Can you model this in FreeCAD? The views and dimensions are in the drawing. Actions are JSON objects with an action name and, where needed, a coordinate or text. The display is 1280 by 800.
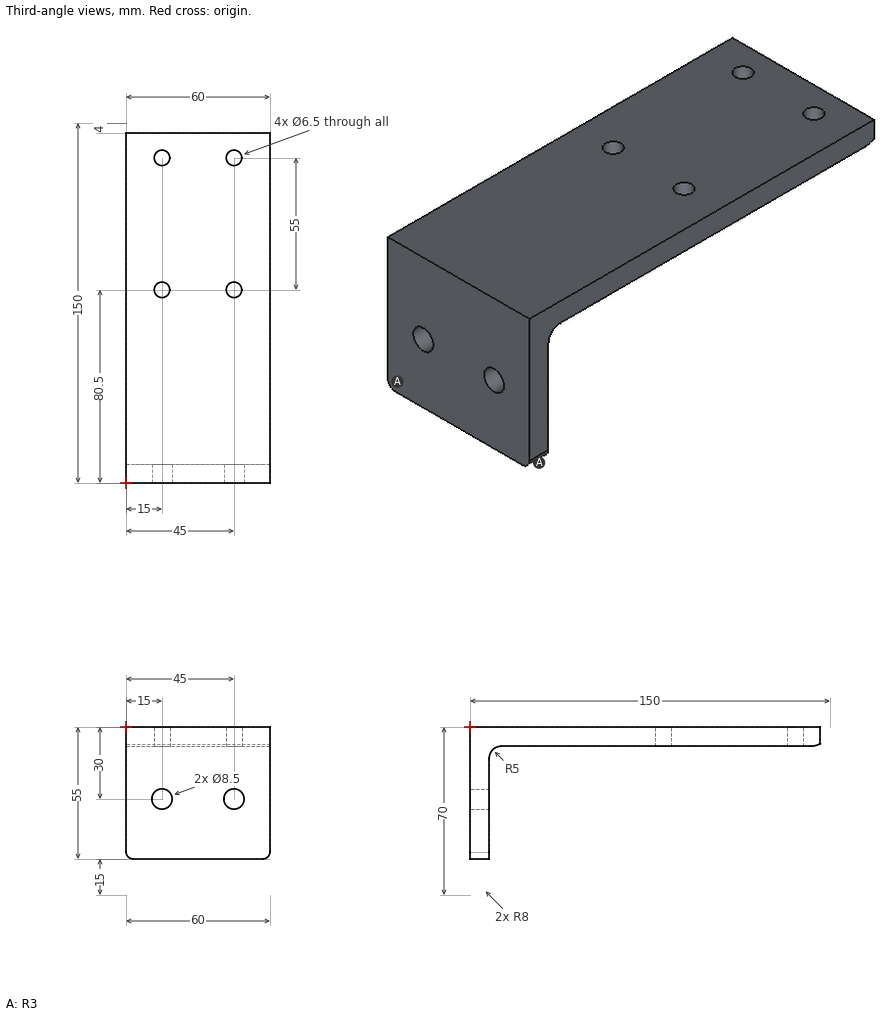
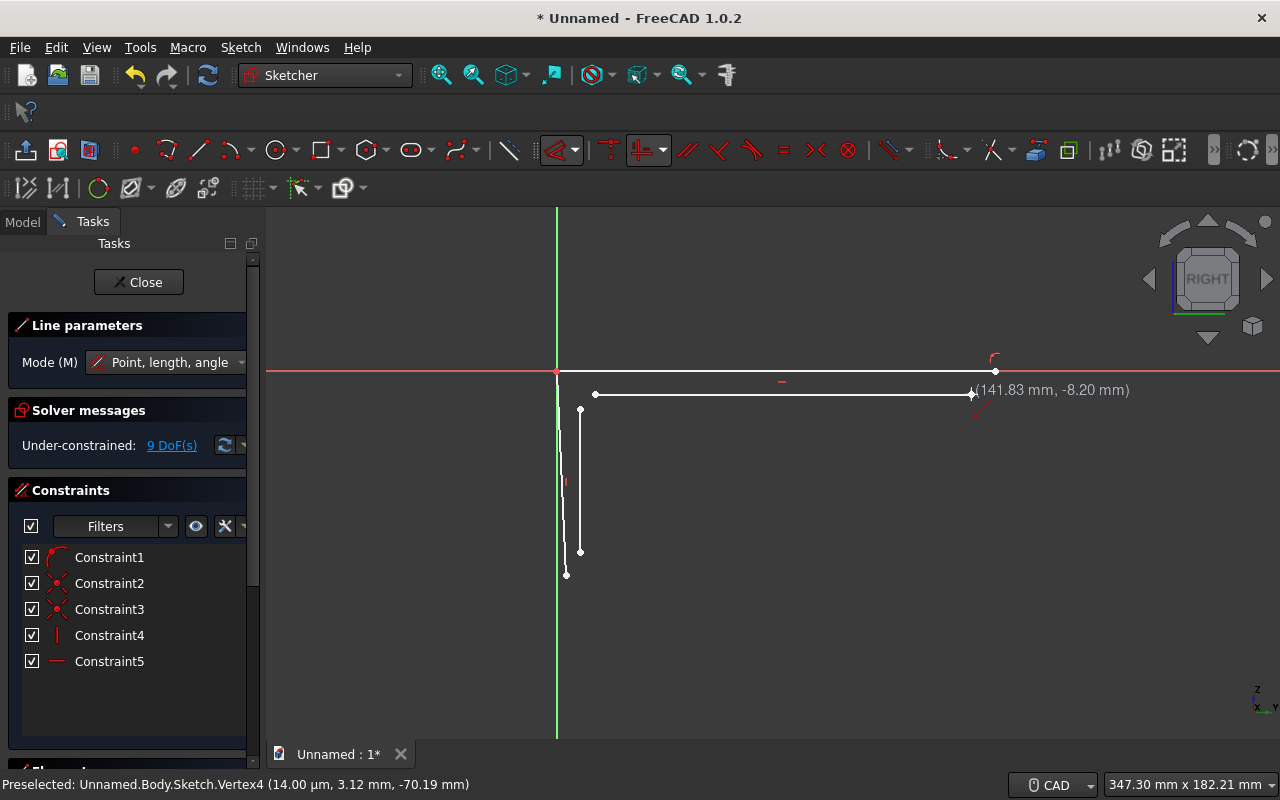
{"action": "key", "text": "g 3 a"}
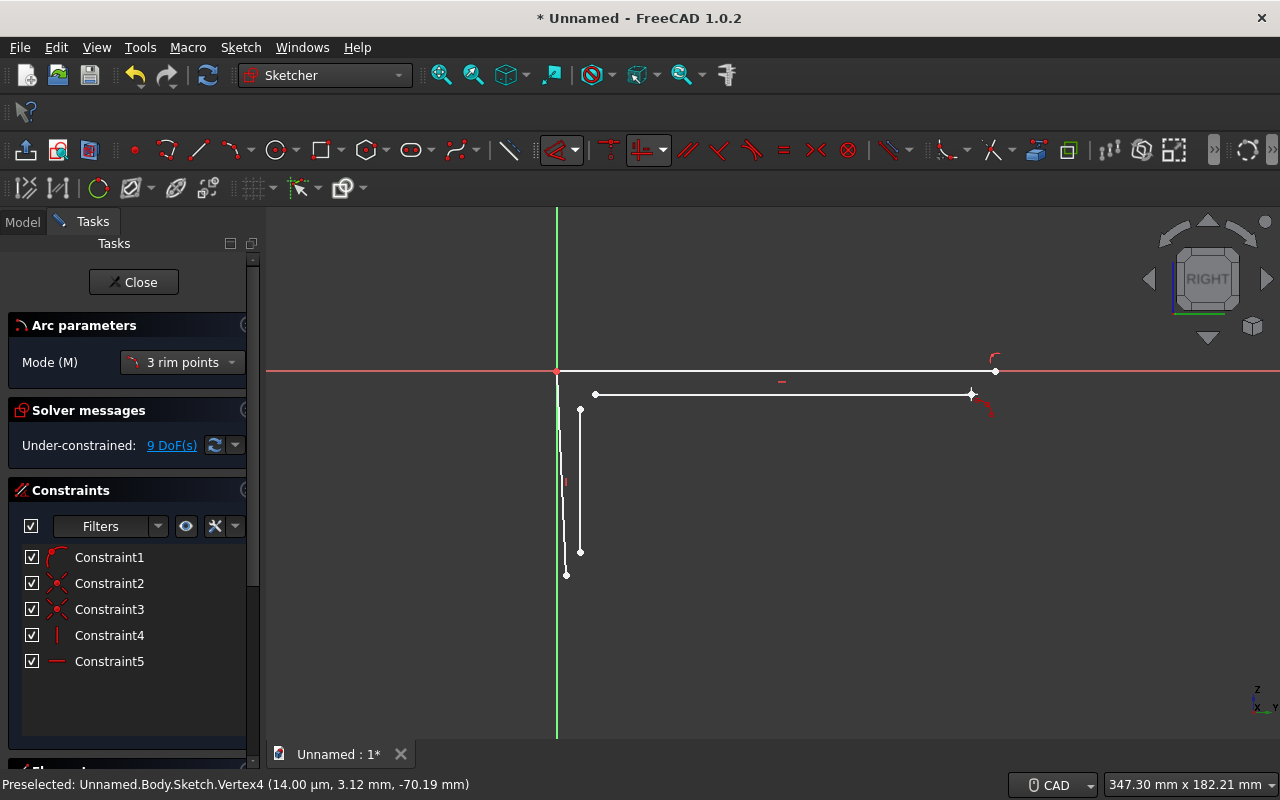
{"action": "left_click", "coordinate": [566, 576]}
{"action": "left_click", "coordinate": [580, 553]}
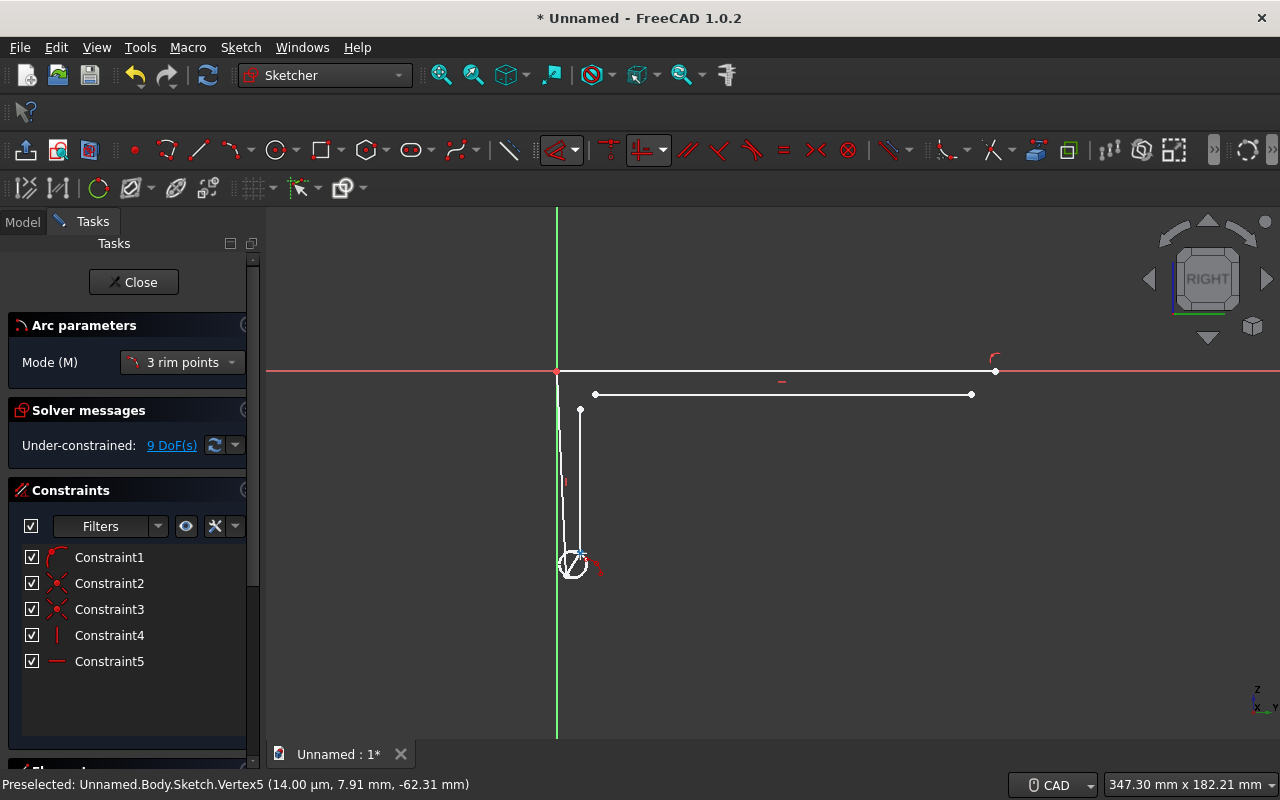
{"action": "scroll", "coordinate": [573, 569], "scroll_direction": "up", "scroll_amount": 5}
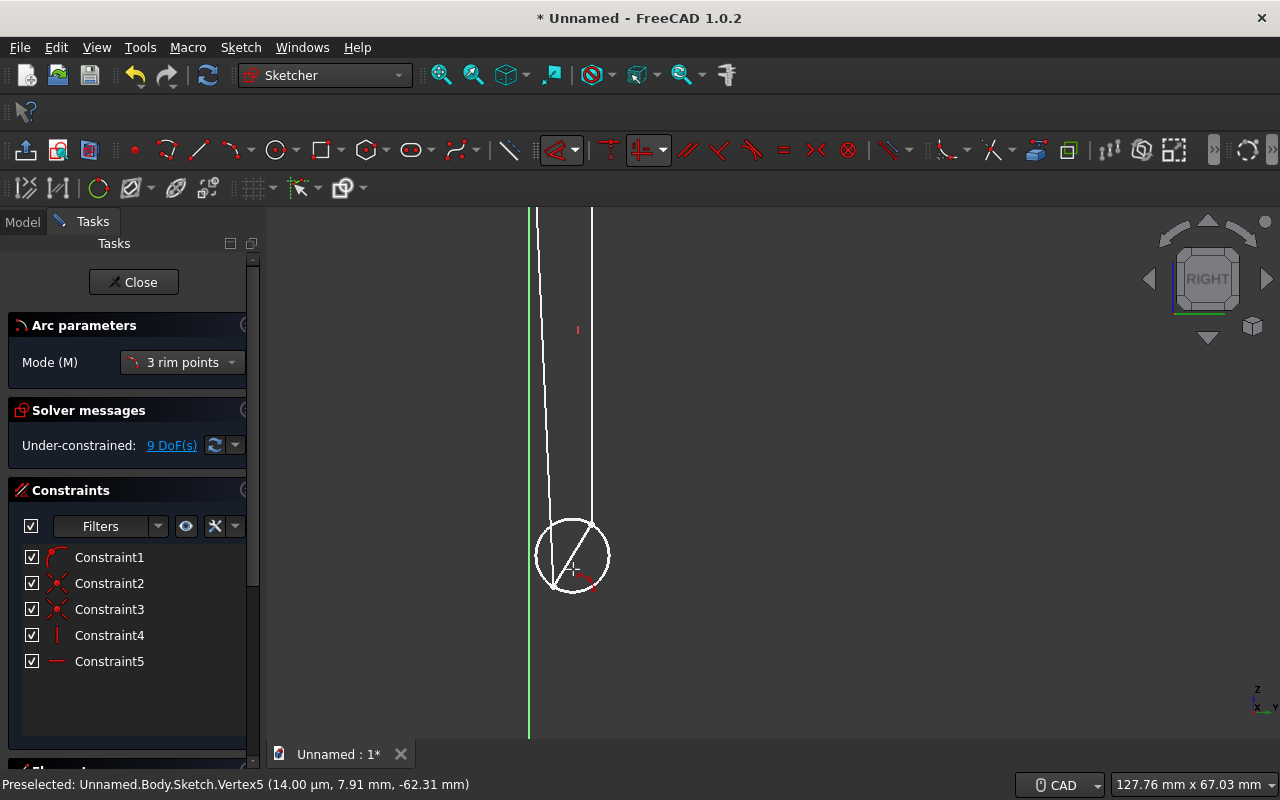
{"action": "left_click", "coordinate": [574, 567]}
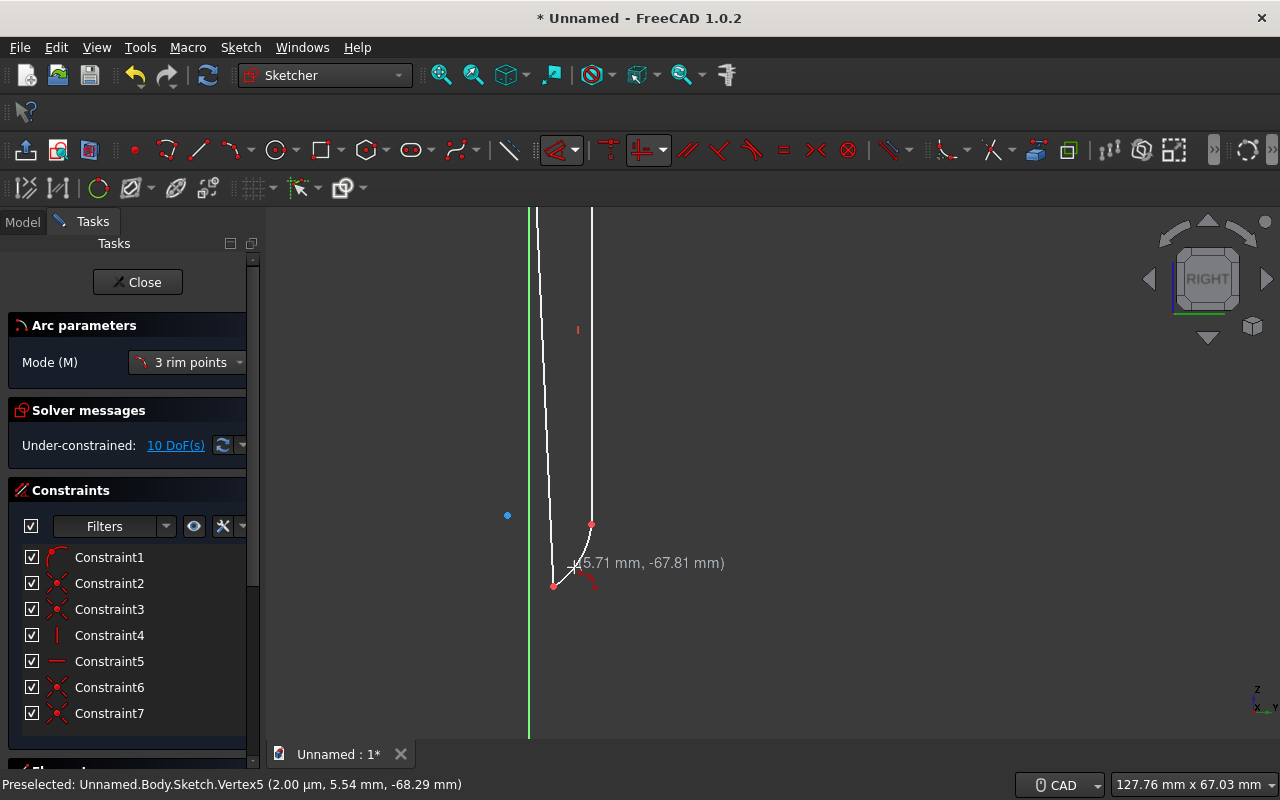
{"action": "scroll", "coordinate": [362, 608], "scroll_direction": "down", "scroll_amount": 4}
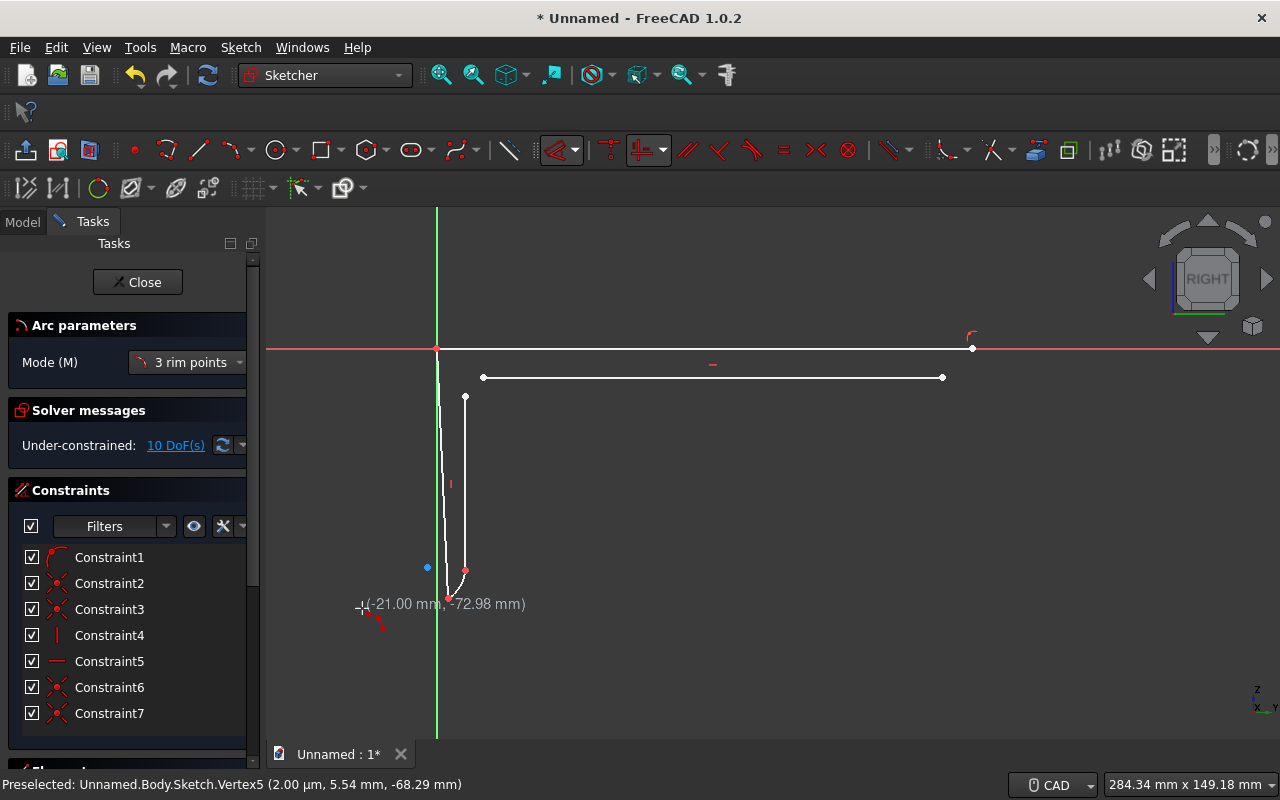
{"action": "left_click", "coordinate": [465, 396]}
{"action": "left_click", "coordinate": [483, 378]}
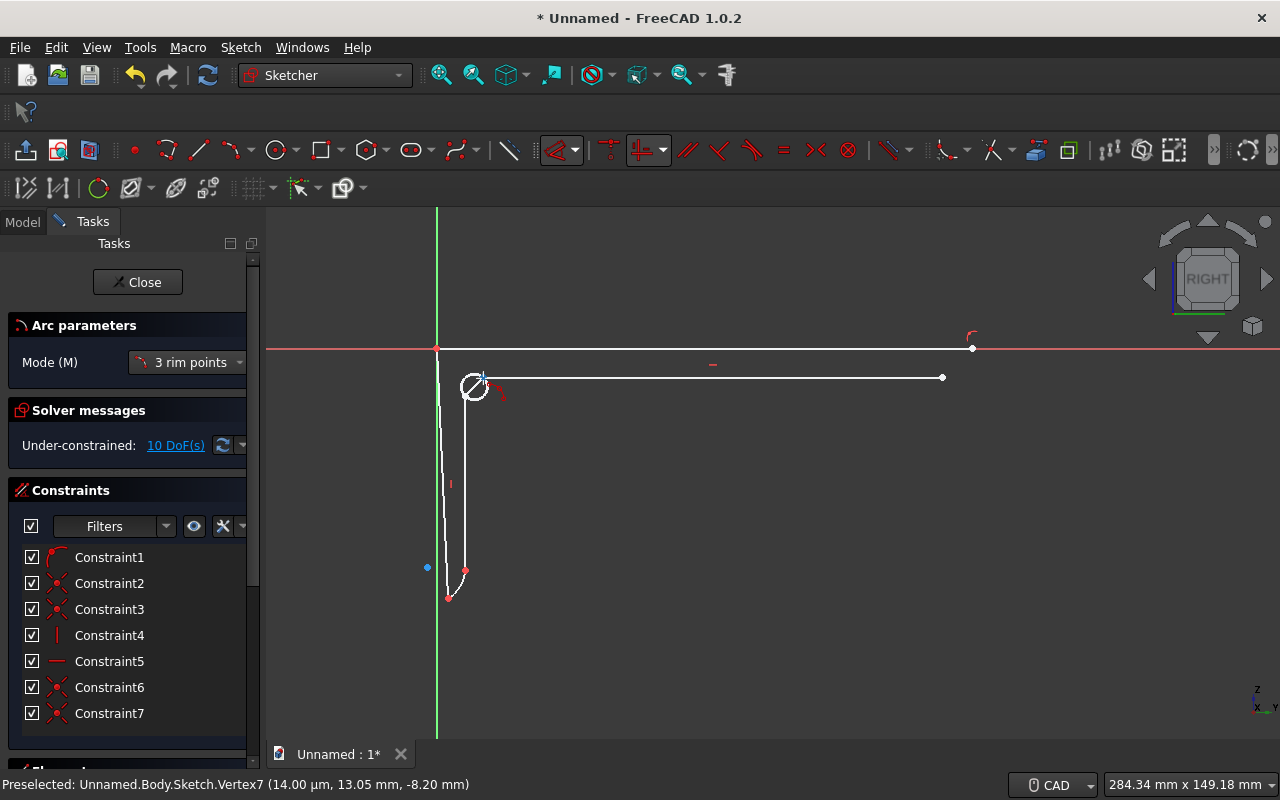
{"action": "scroll", "coordinate": [471, 382], "scroll_direction": "up", "scroll_amount": 6}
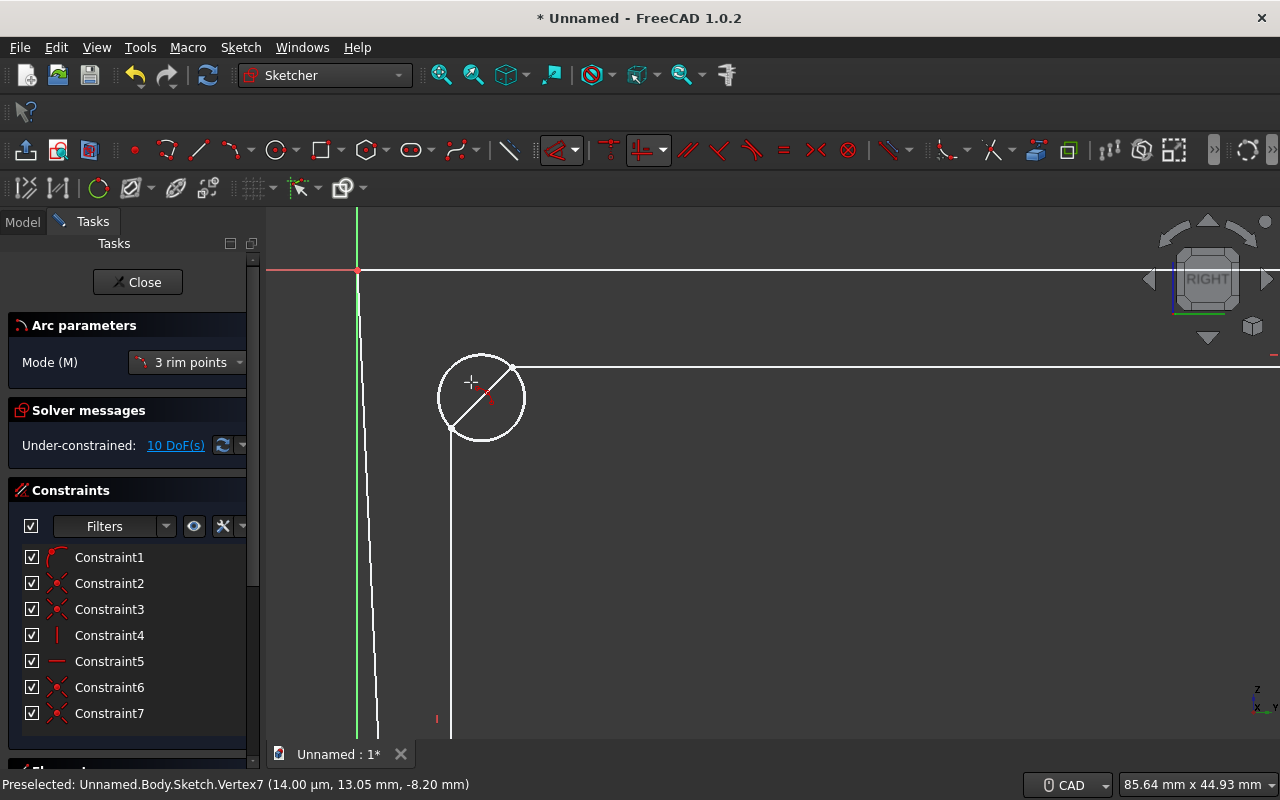
{"action": "left_click", "coordinate": [470, 382]}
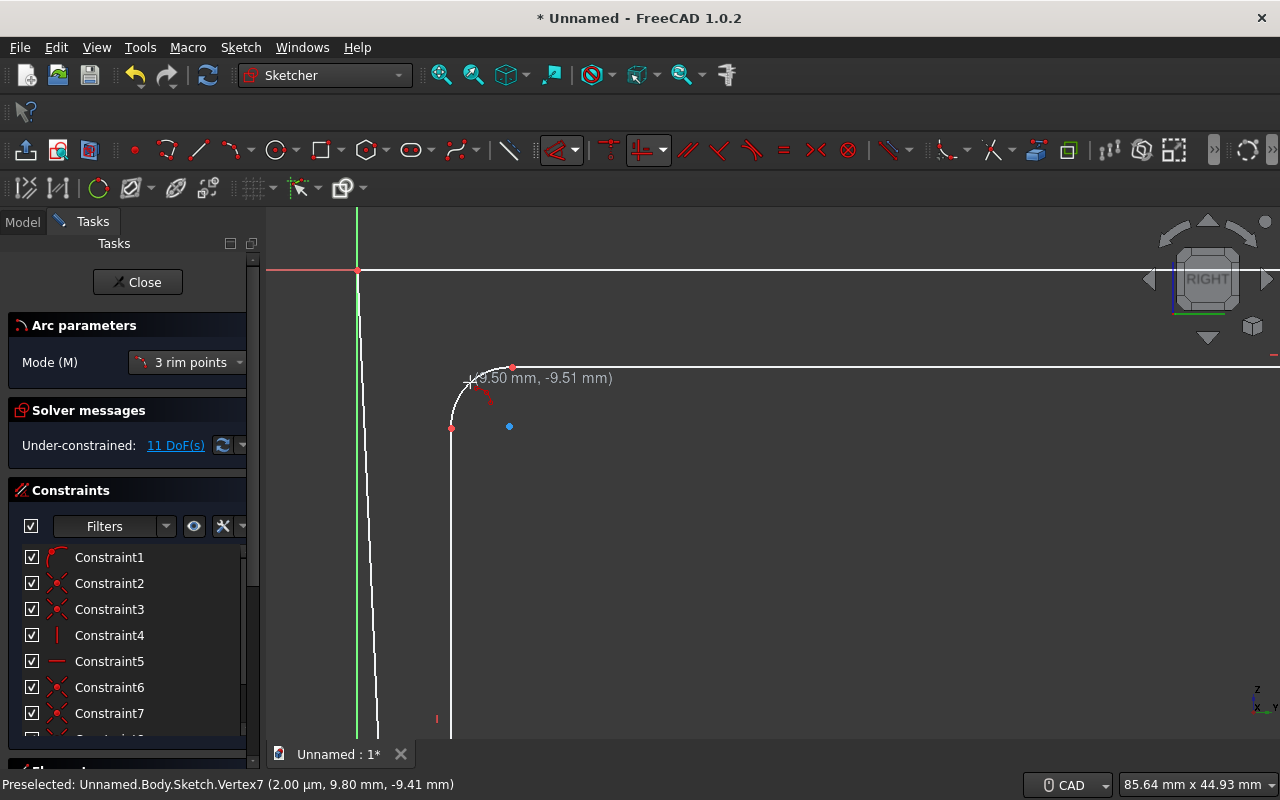
{"action": "scroll", "coordinate": [471, 382], "scroll_direction": "down", "scroll_amount": 6}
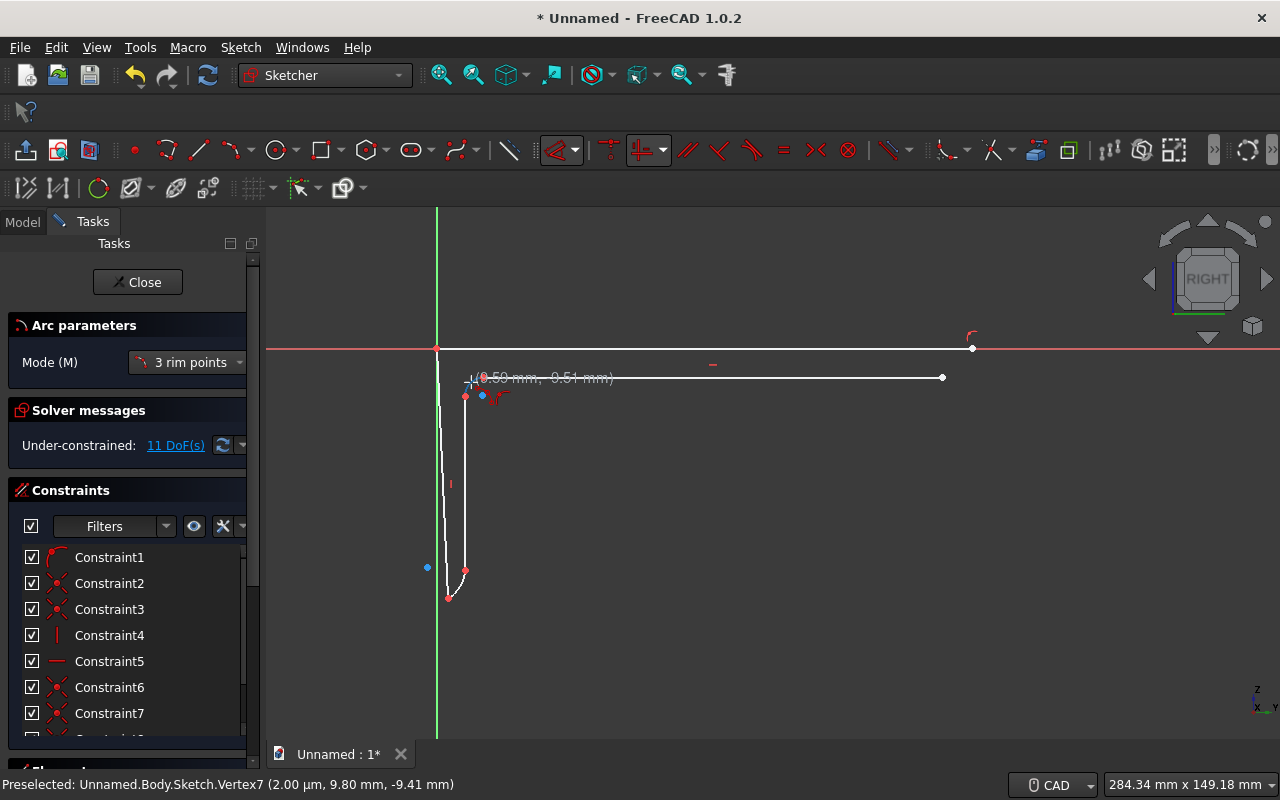
{"action": "left_click", "coordinate": [943, 378]}
{"action": "left_click", "coordinate": [972, 349]}